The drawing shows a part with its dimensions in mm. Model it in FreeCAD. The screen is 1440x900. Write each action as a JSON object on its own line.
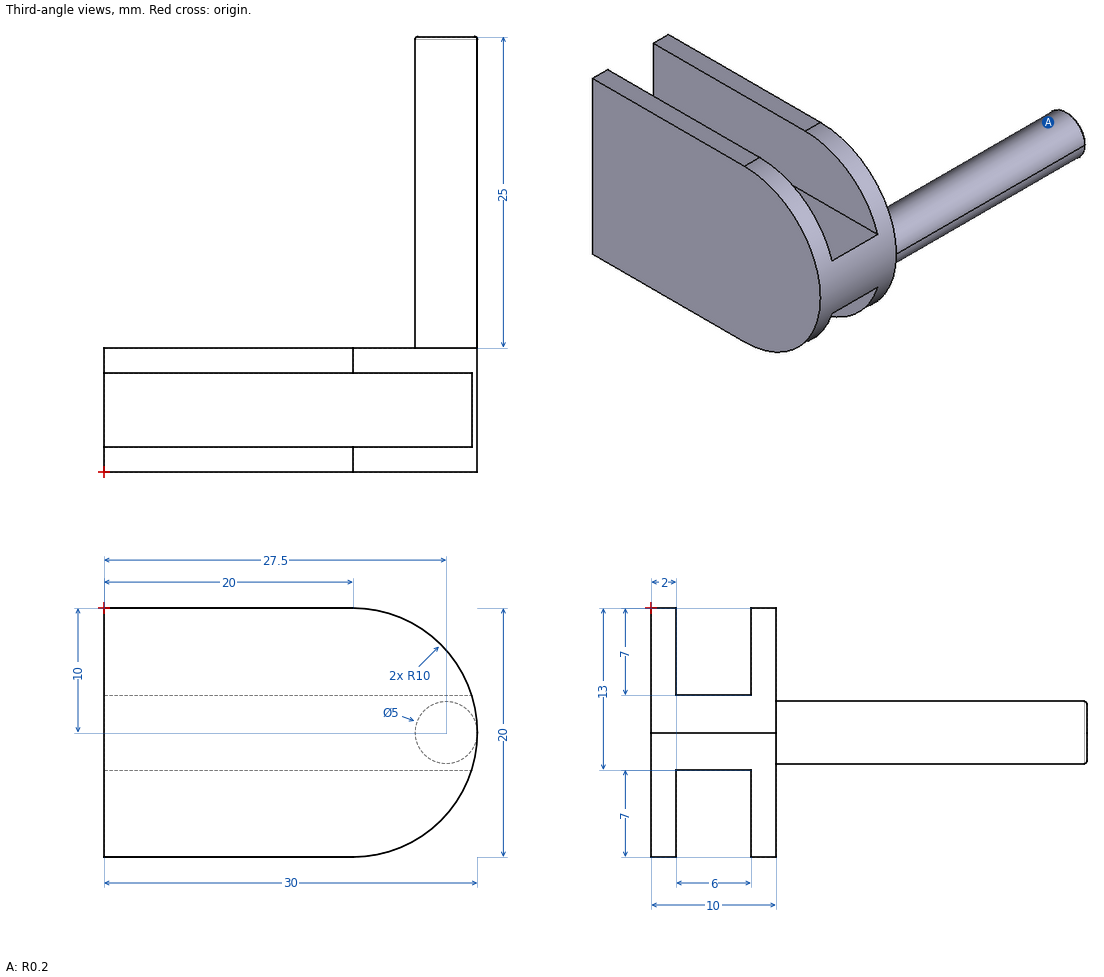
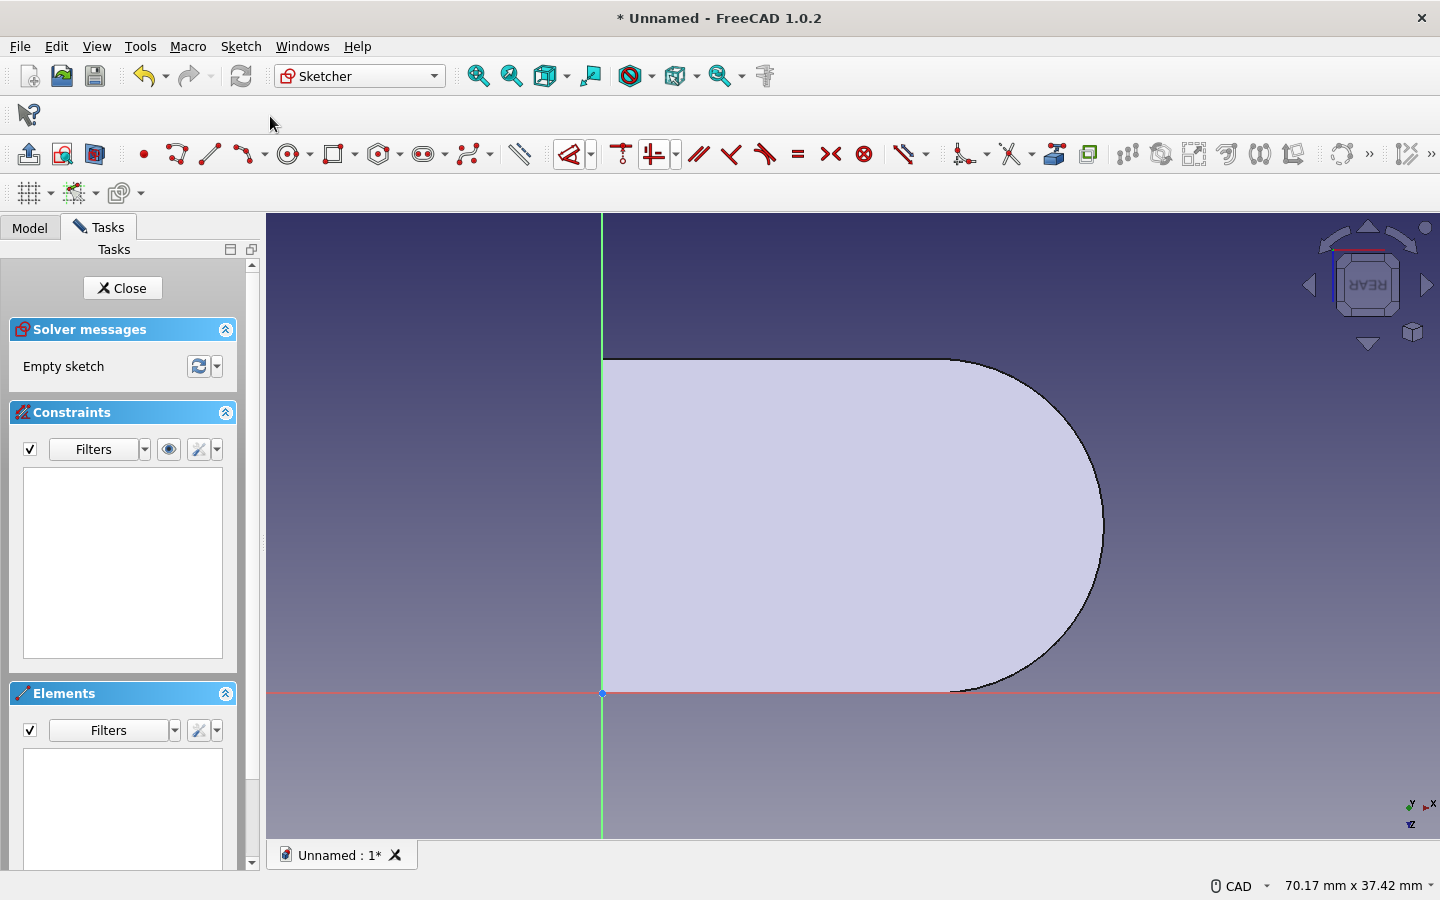
{"action": "scroll", "coordinate": [1132, 526], "scroll_direction": "up", "scroll_amount": 8}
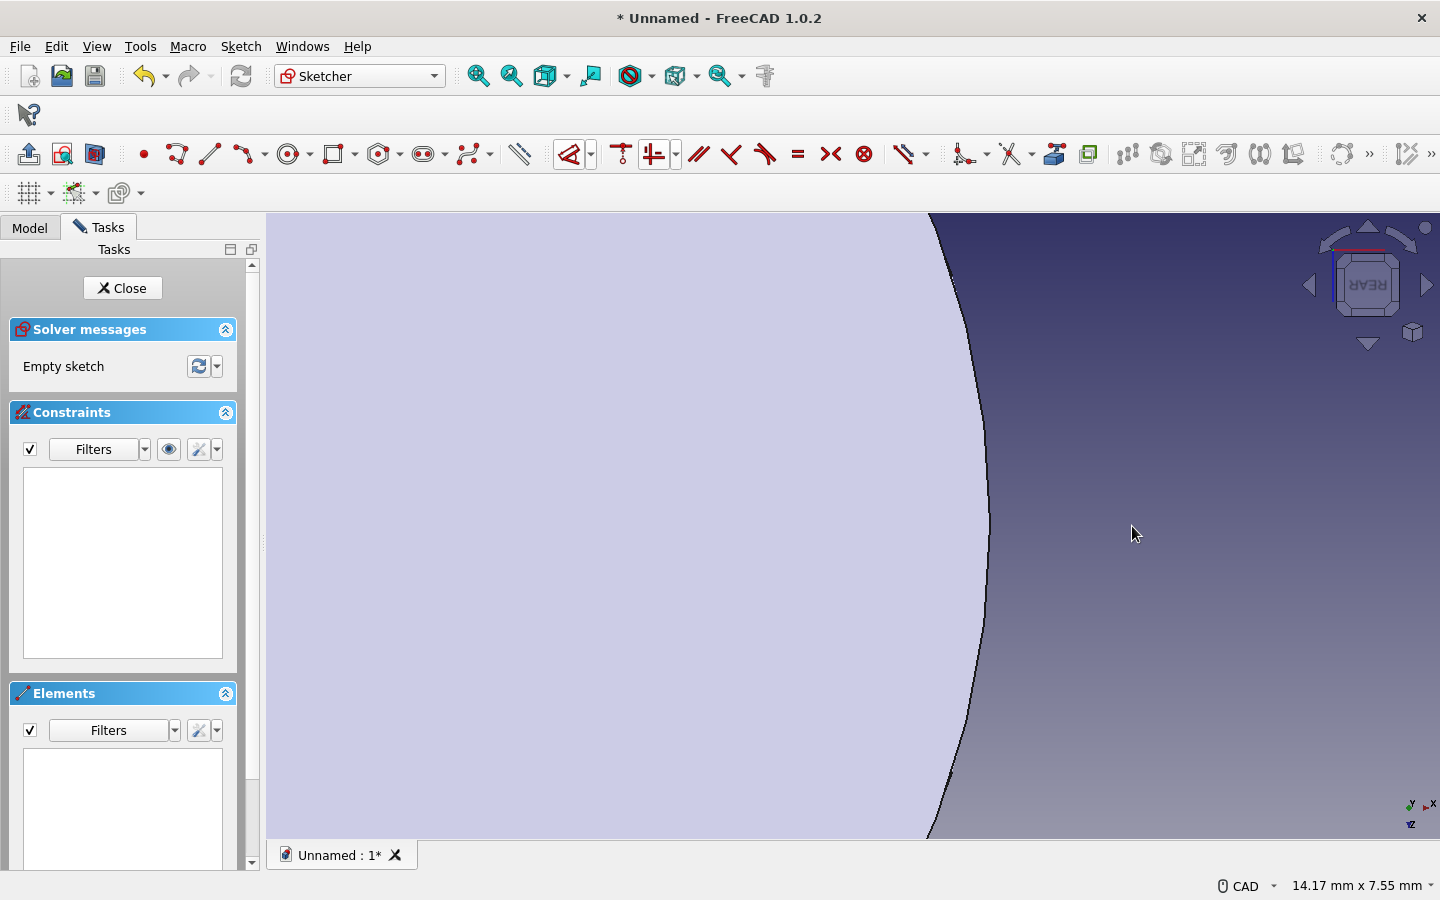
{"action": "left_click", "coordinate": [288, 154]}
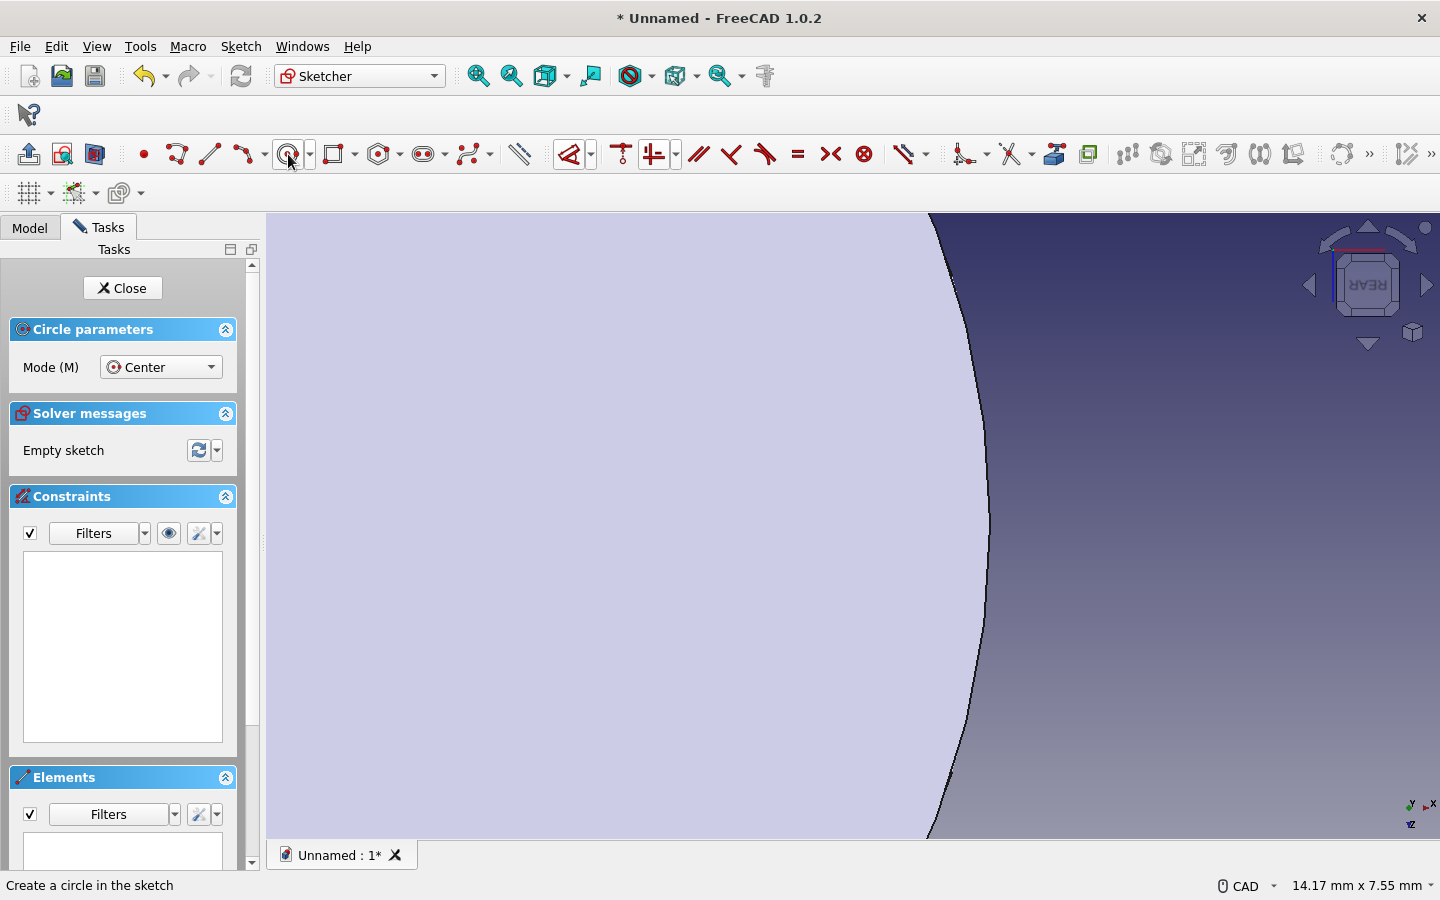
{"action": "left_click", "coordinate": [783, 524]}
{"action": "mouse_move", "coordinate": [930, 378]}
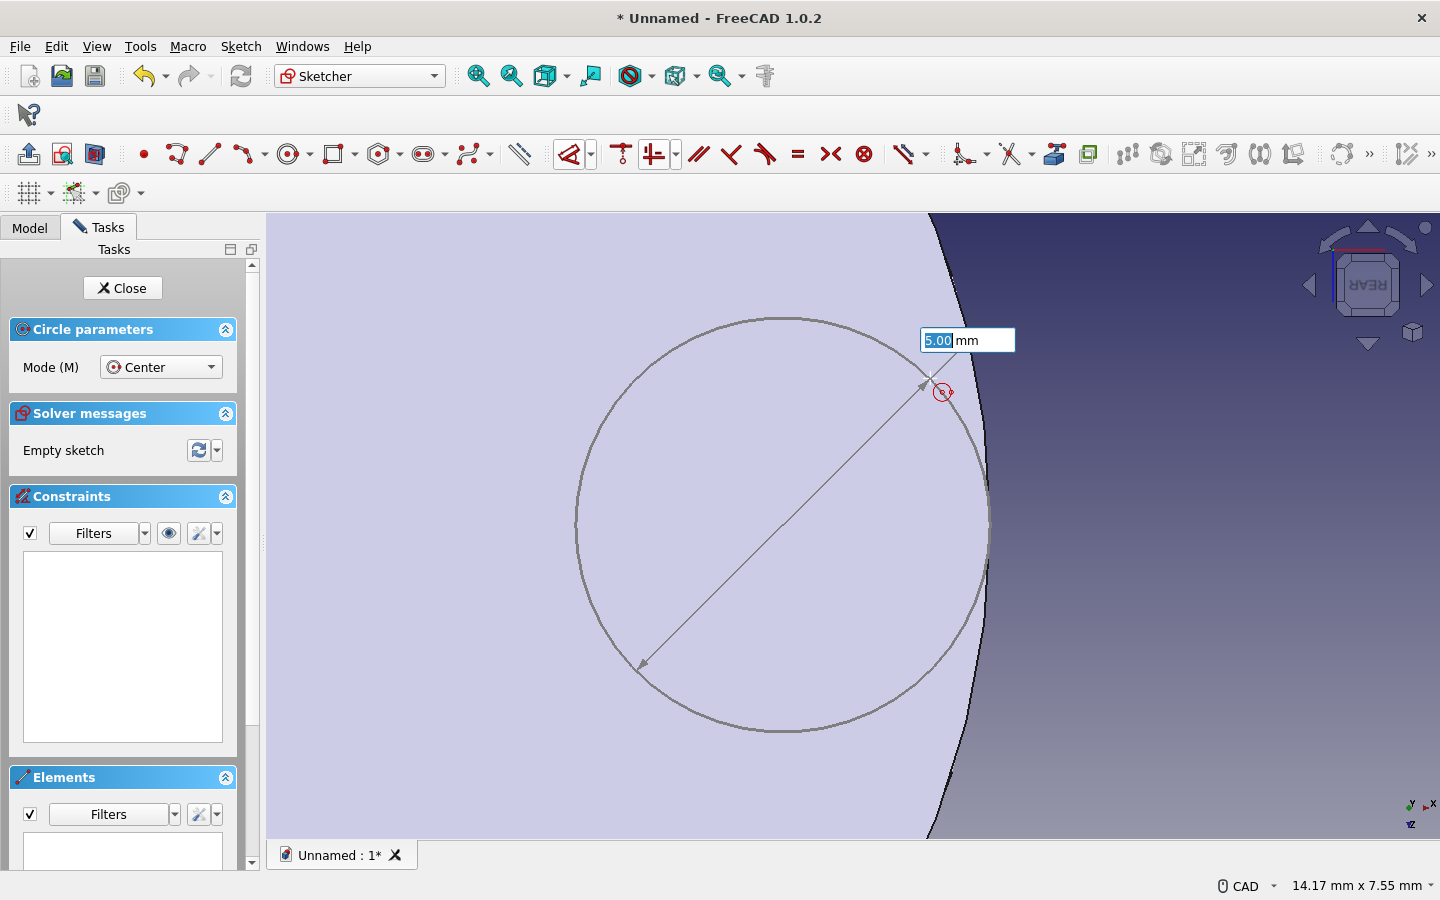
{"action": "type", "text": "5"}
{"action": "key", "text": "Return"}
{"action": "key", "text": "Escape"}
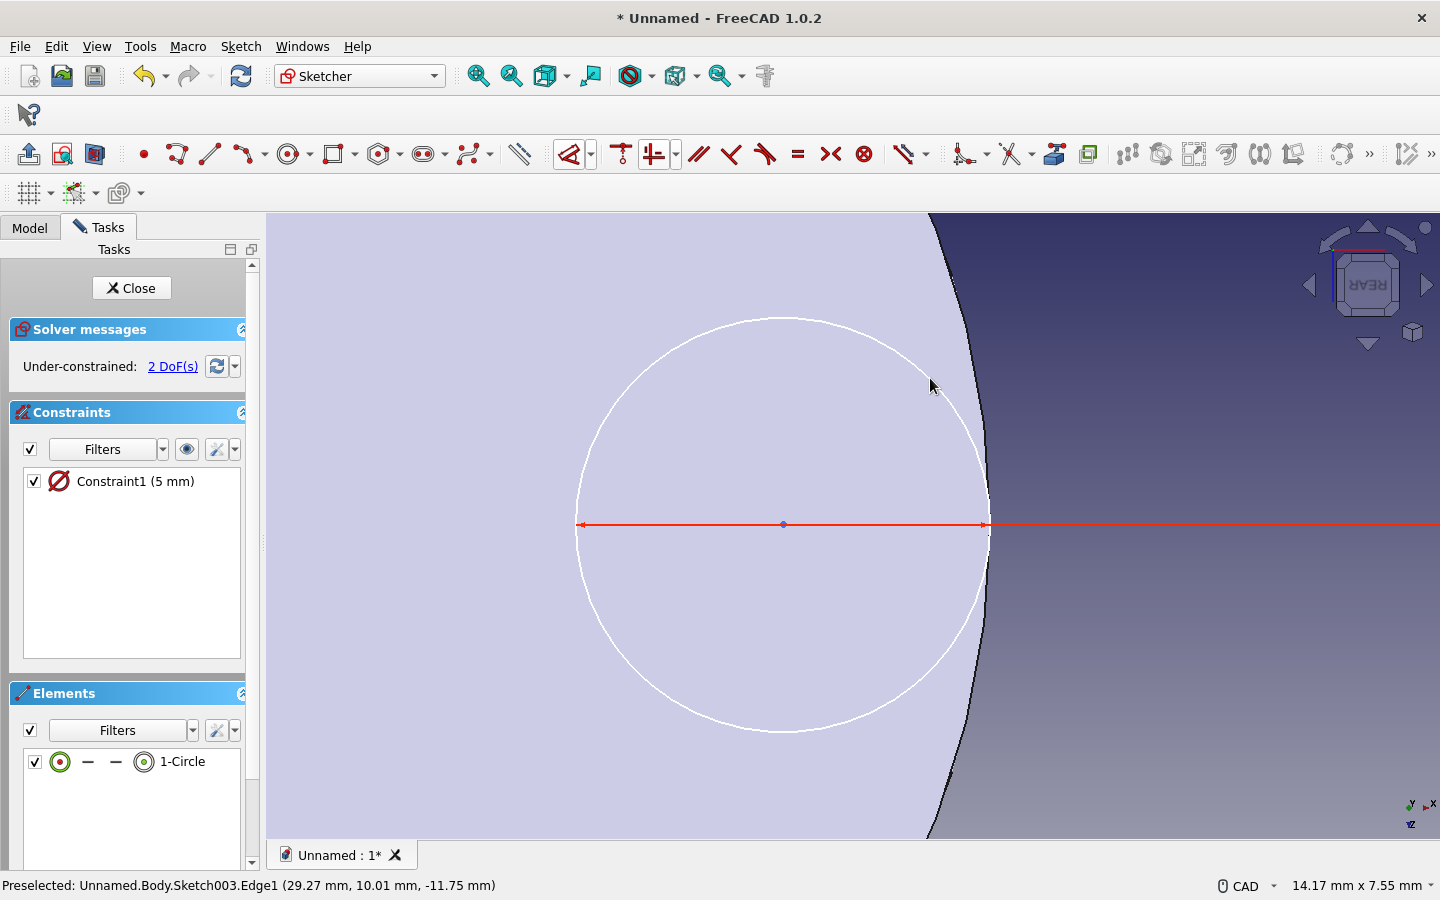
{"action": "left_click", "coordinate": [783, 525]}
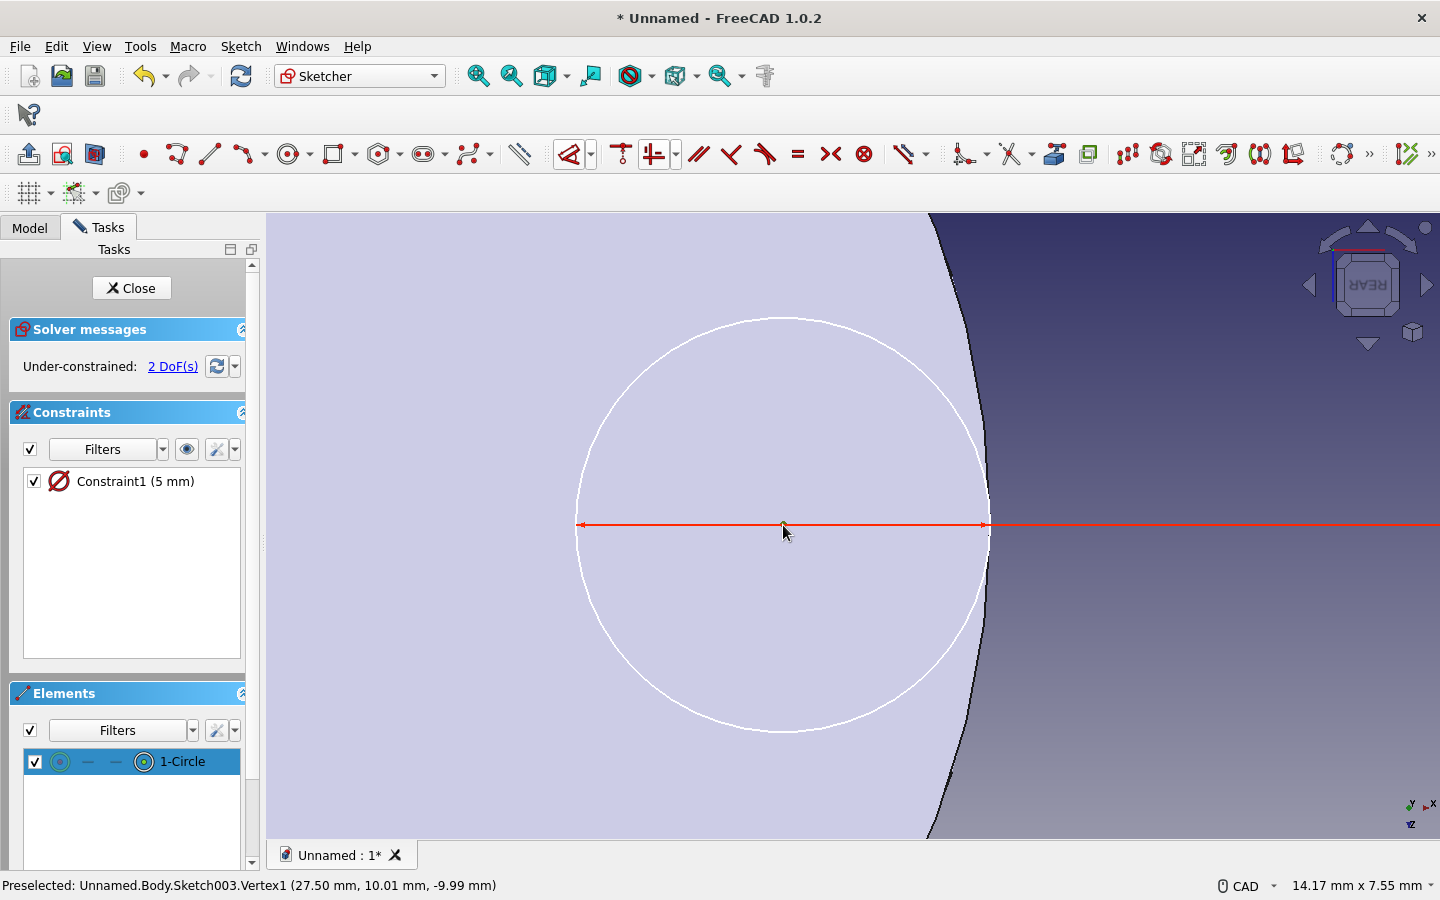
{"action": "key", "text": "i"}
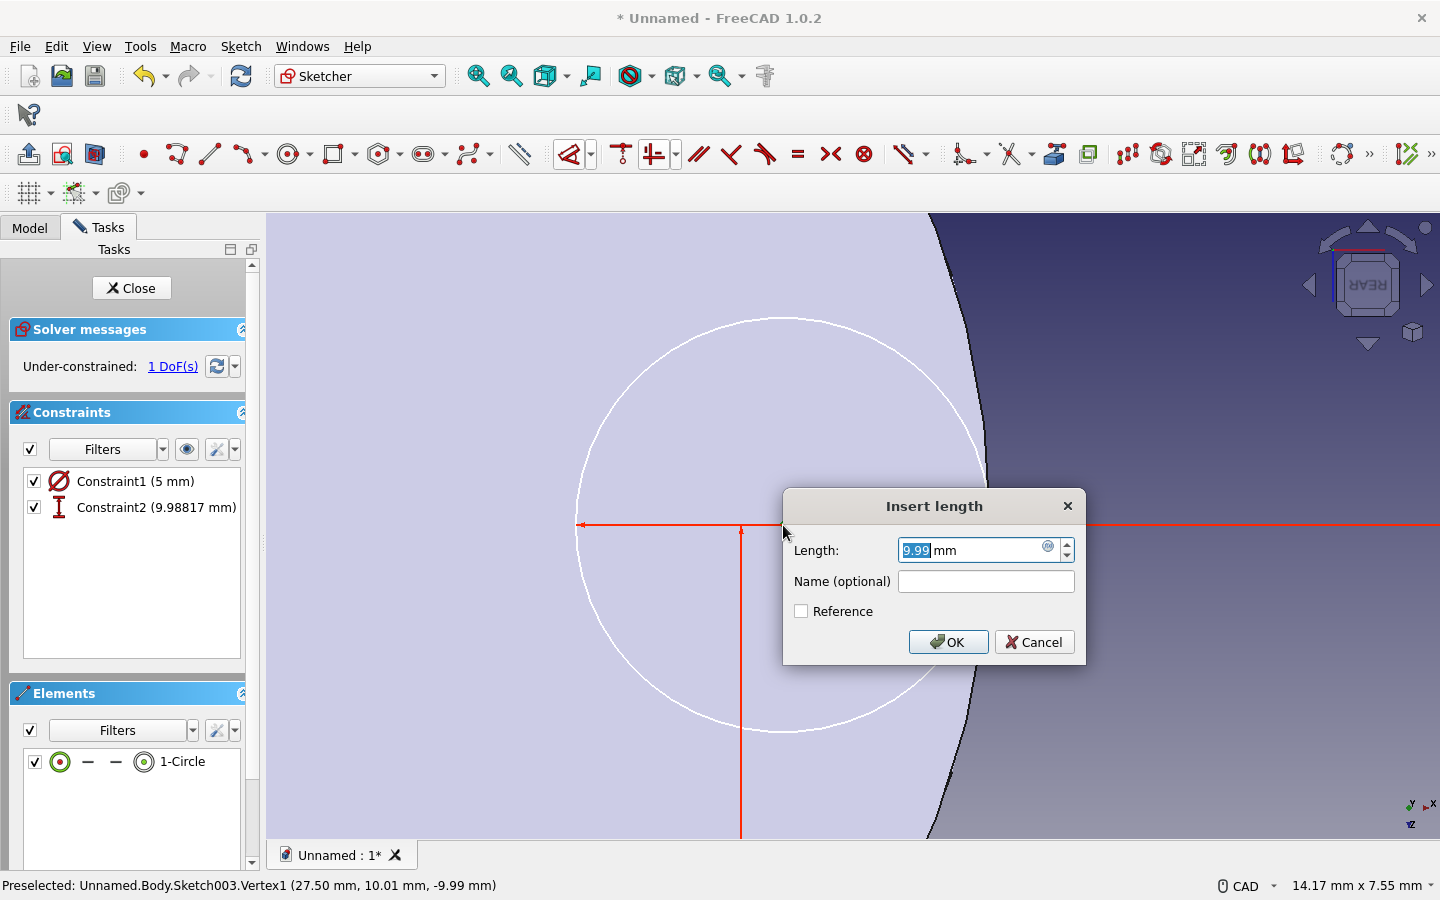
{"action": "type", "text": "10"}
{"action": "key", "text": "Return"}